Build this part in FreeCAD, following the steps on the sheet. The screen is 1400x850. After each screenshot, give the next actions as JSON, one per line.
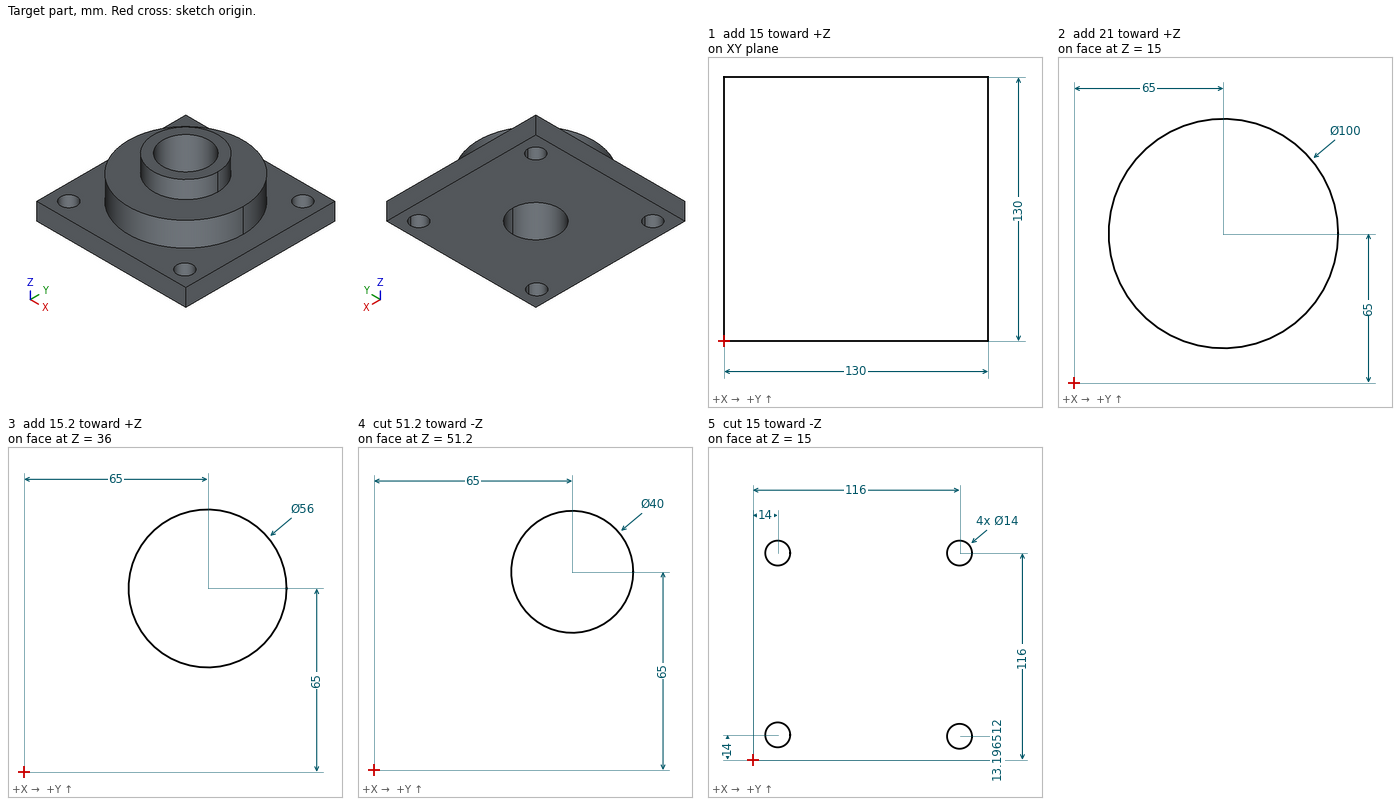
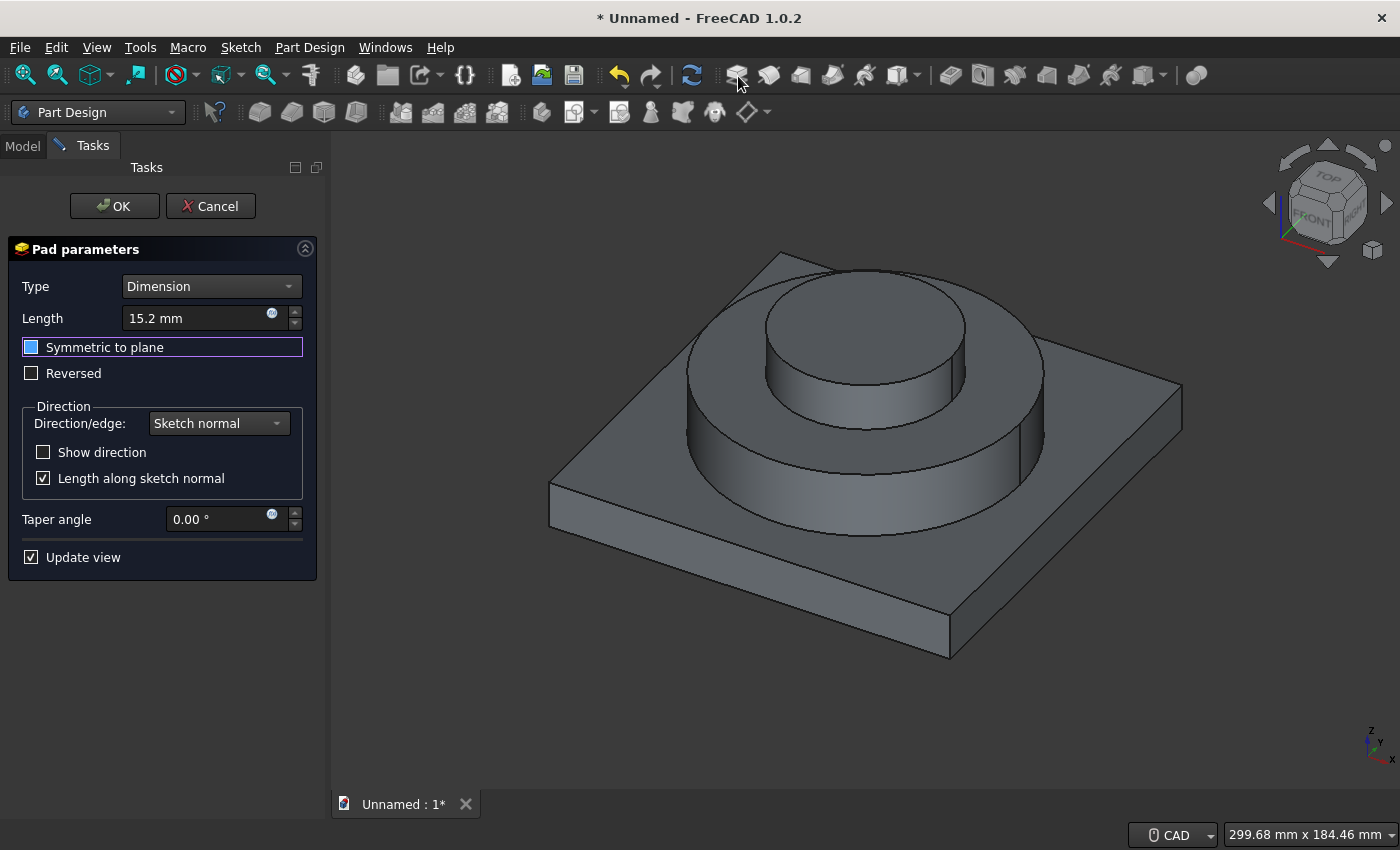
{"action": "left_click", "coordinate": [115, 206]}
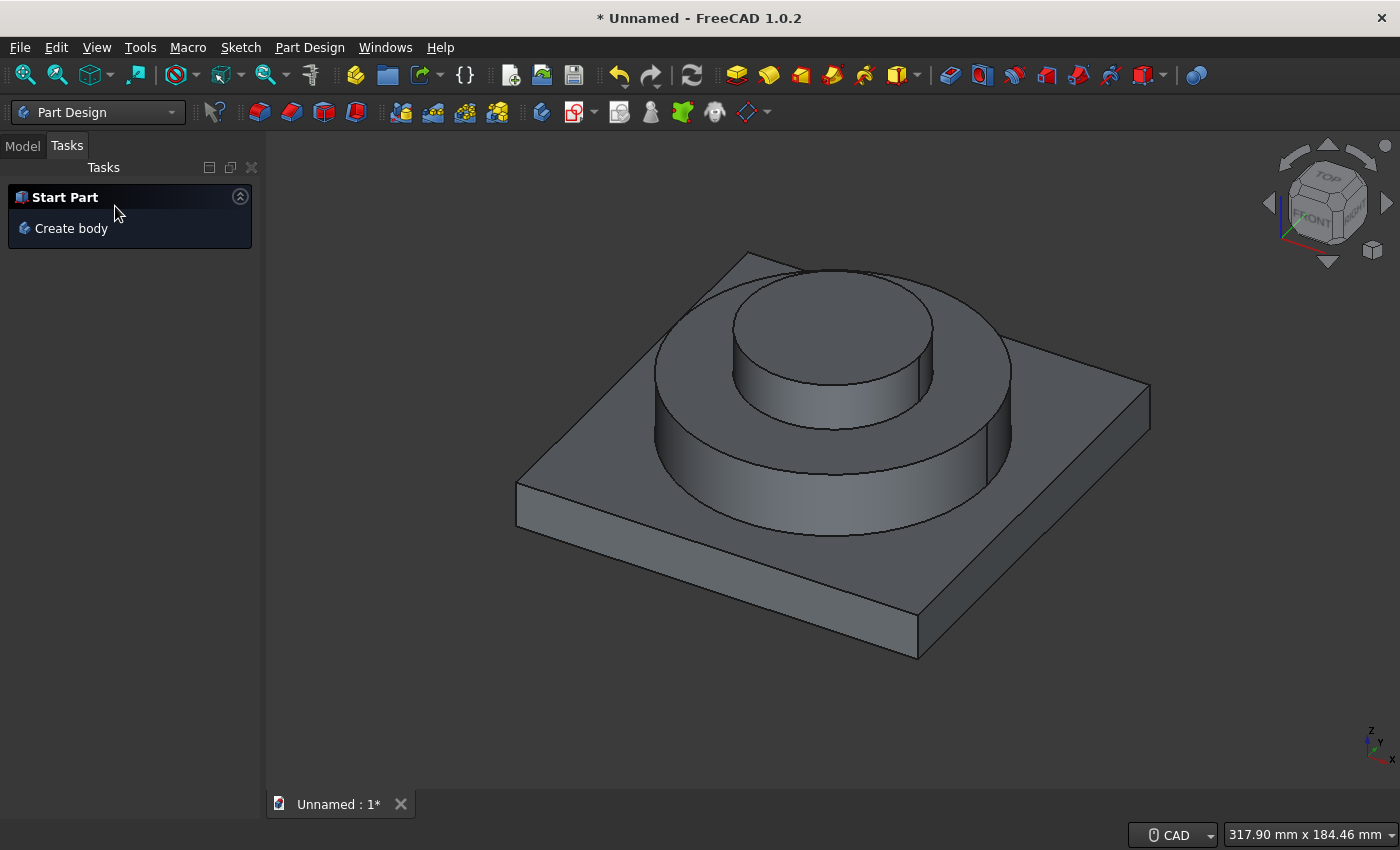
{"action": "left_click", "coordinate": [833, 327]}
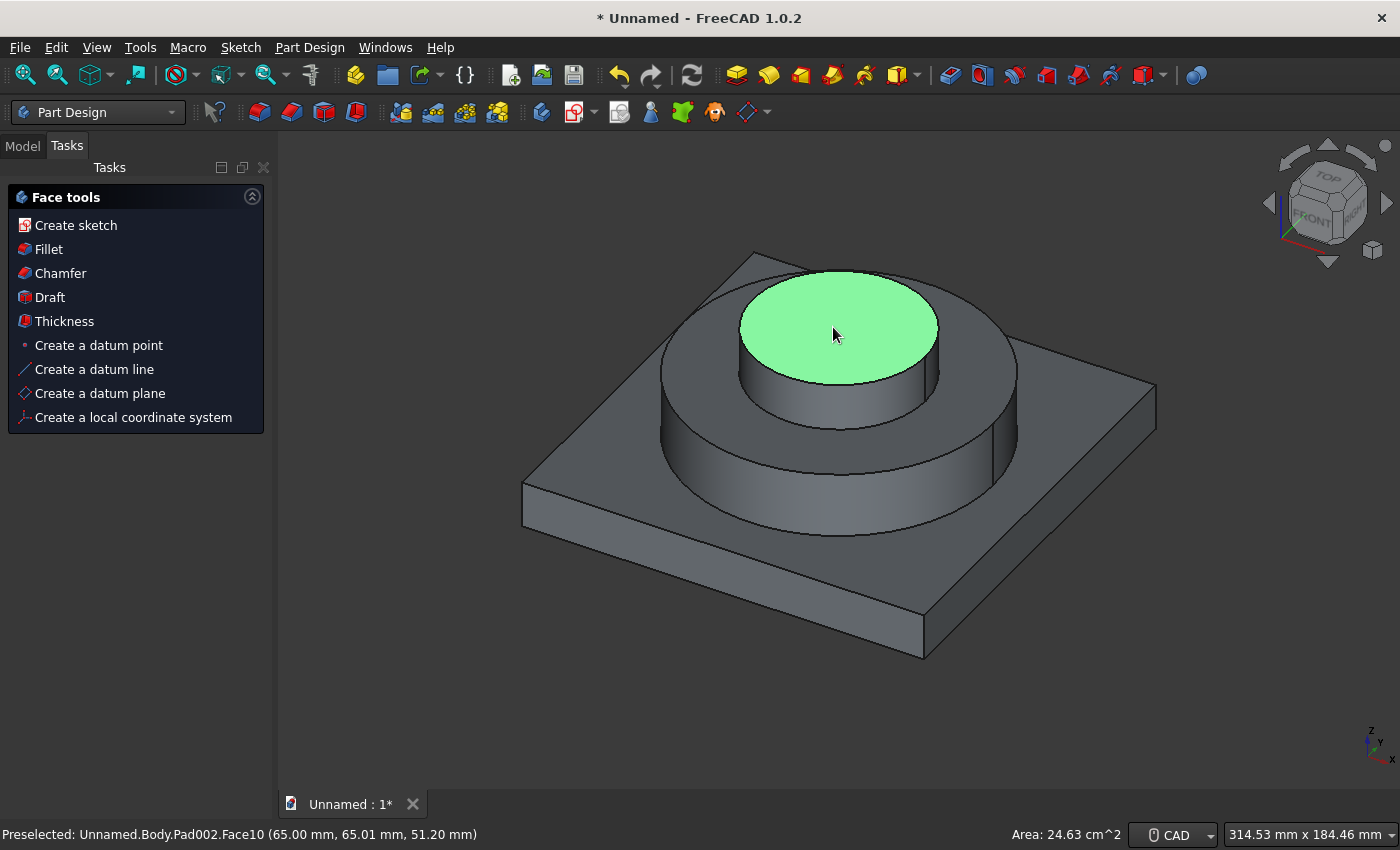
{"action": "left_click", "coordinate": [574, 112]}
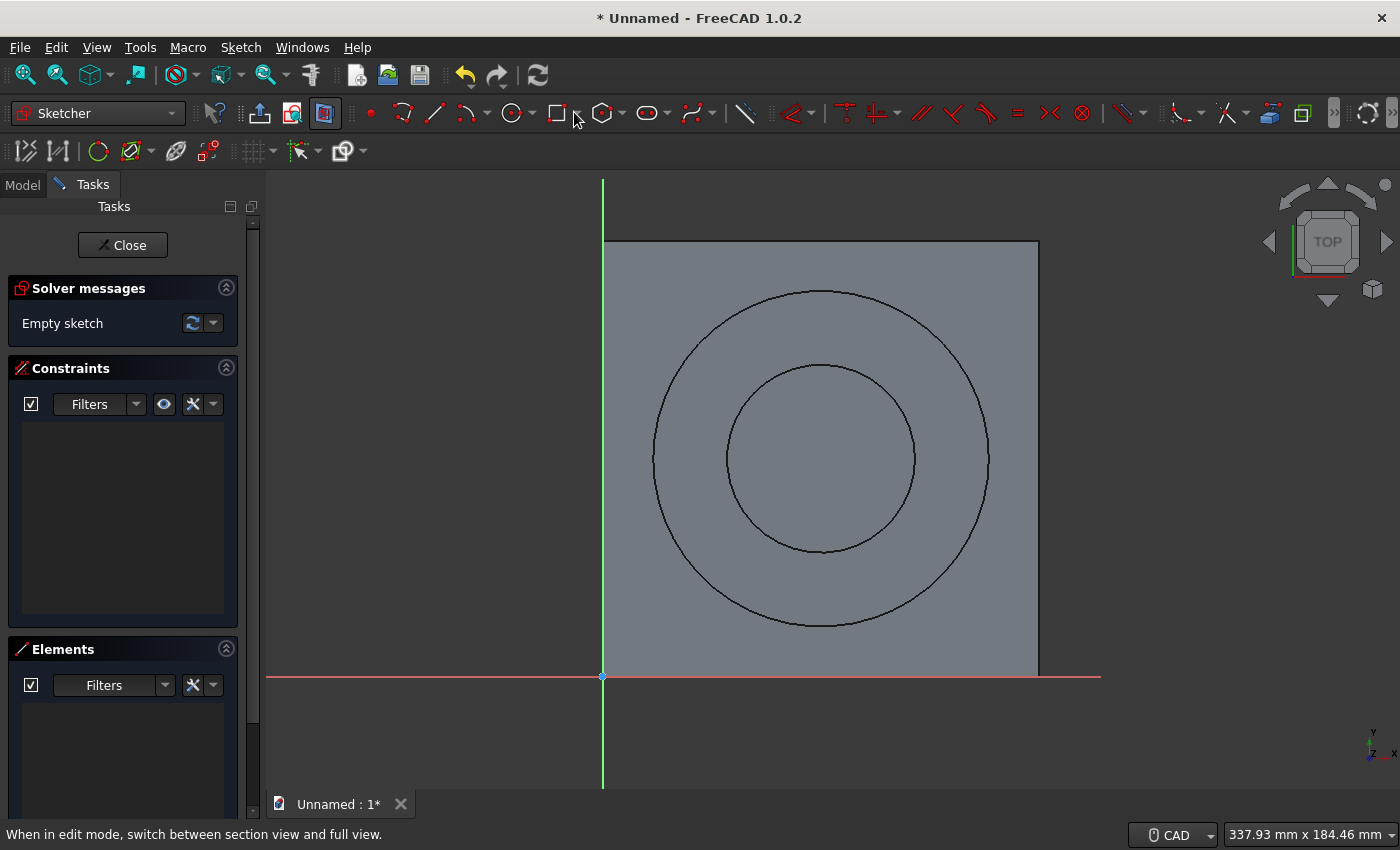
{"action": "scroll", "coordinate": [707, 646], "scroll_direction": "up", "scroll_amount": 2}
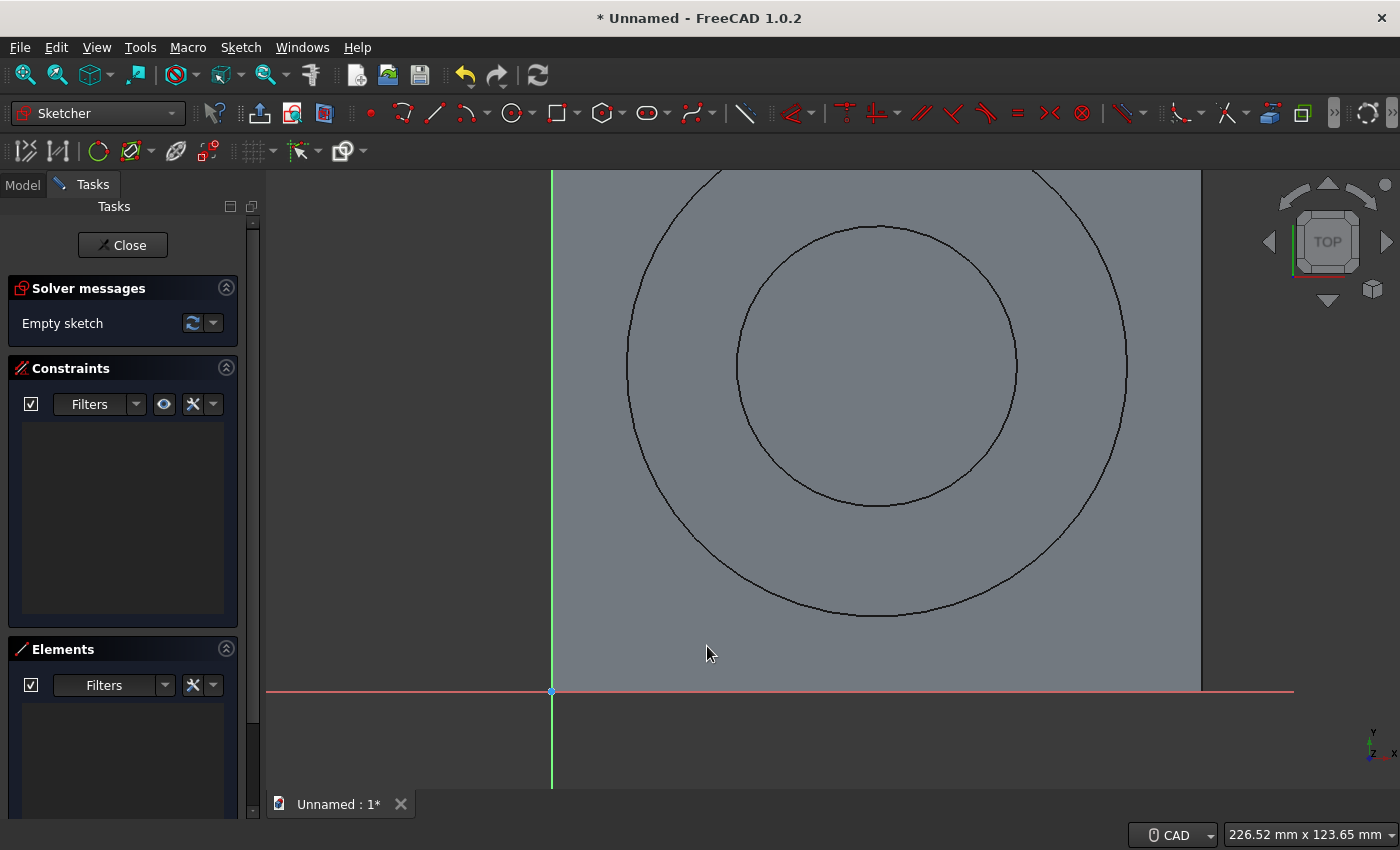
{"action": "key", "text": "g c"}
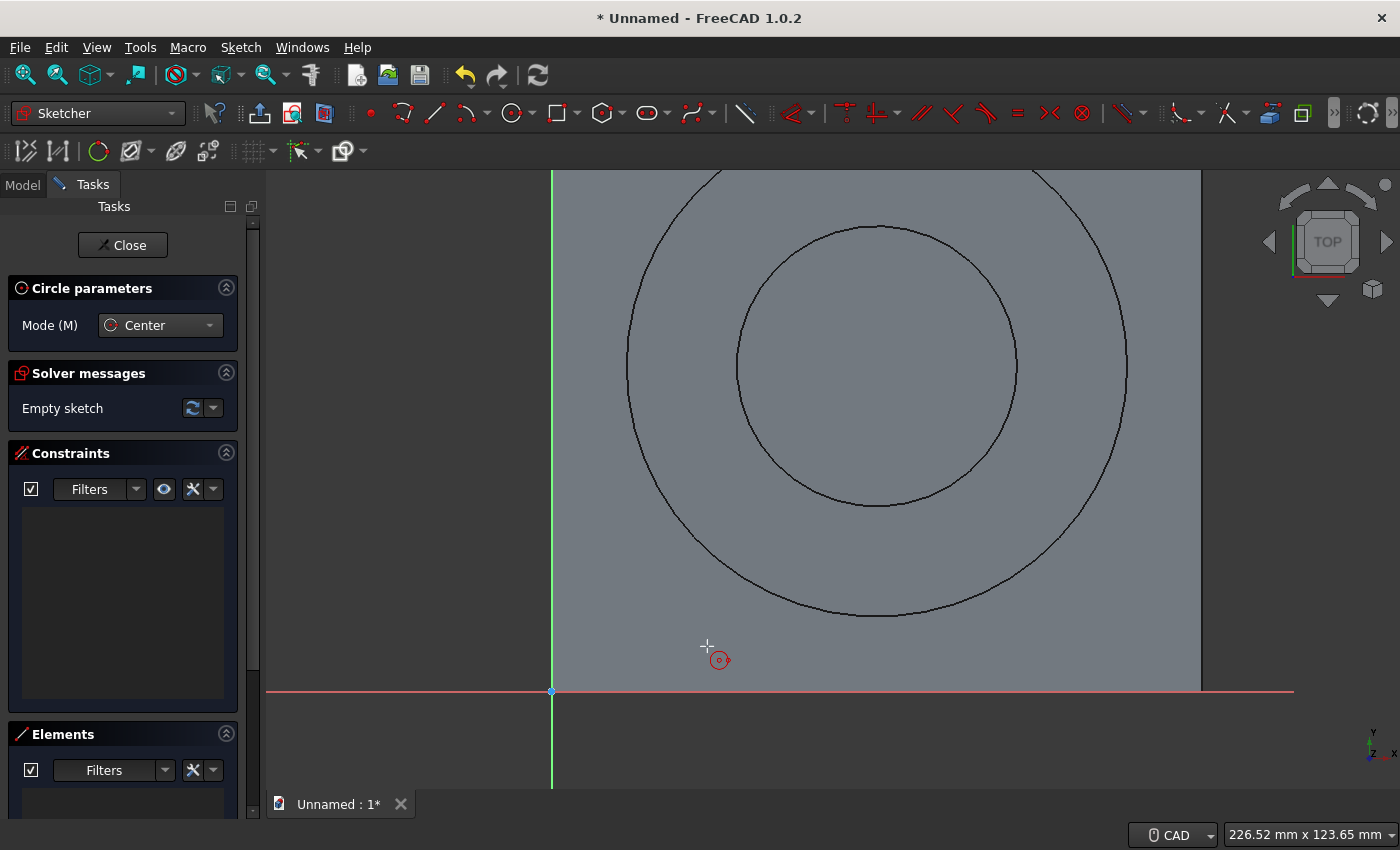
{"action": "left_click", "coordinate": [877, 366]}
{"action": "mouse_move", "coordinate": [948, 296]}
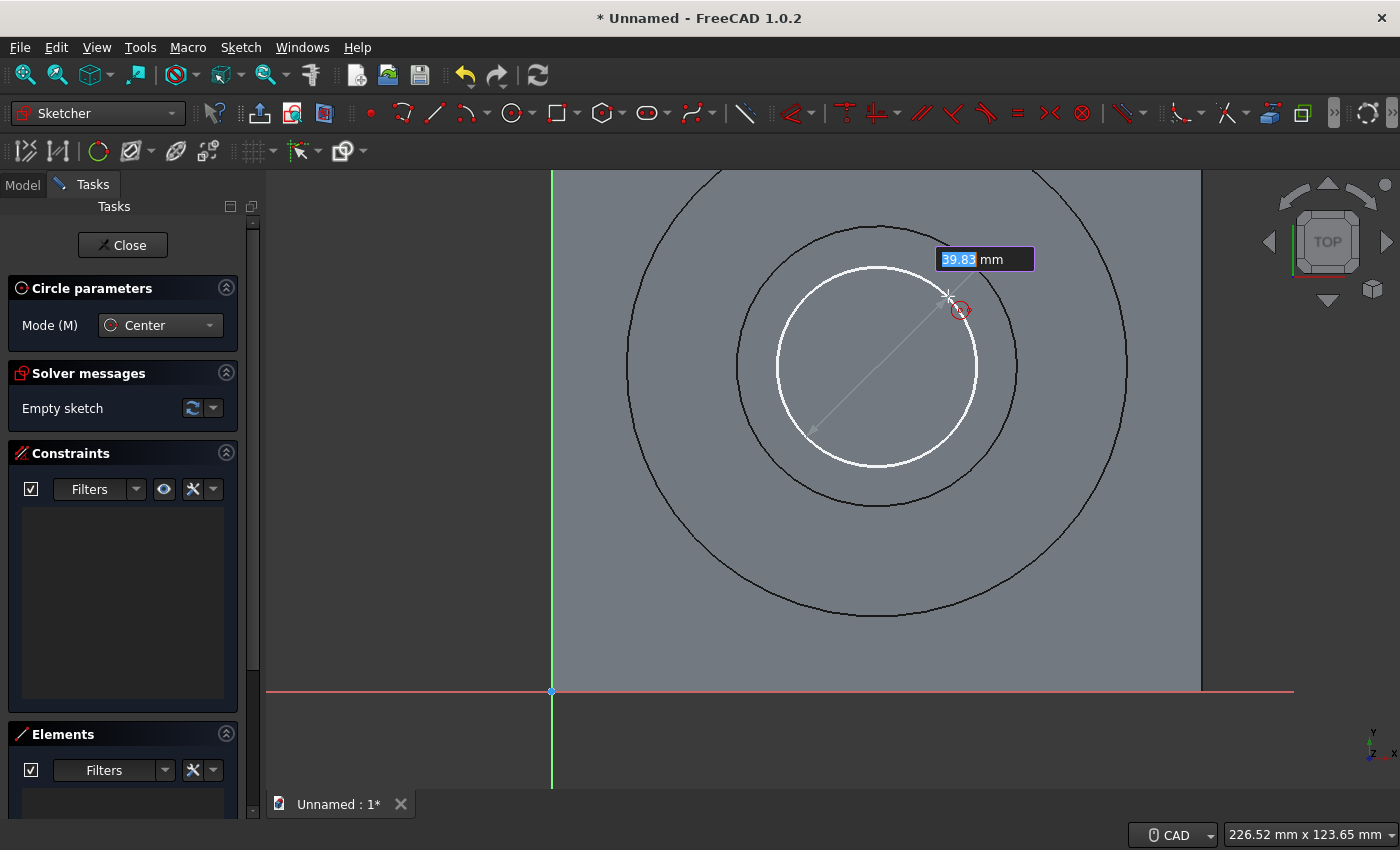
{"action": "type", "text": "40"}
{"action": "key", "text": "Return"}
{"action": "key", "text": "Escape"}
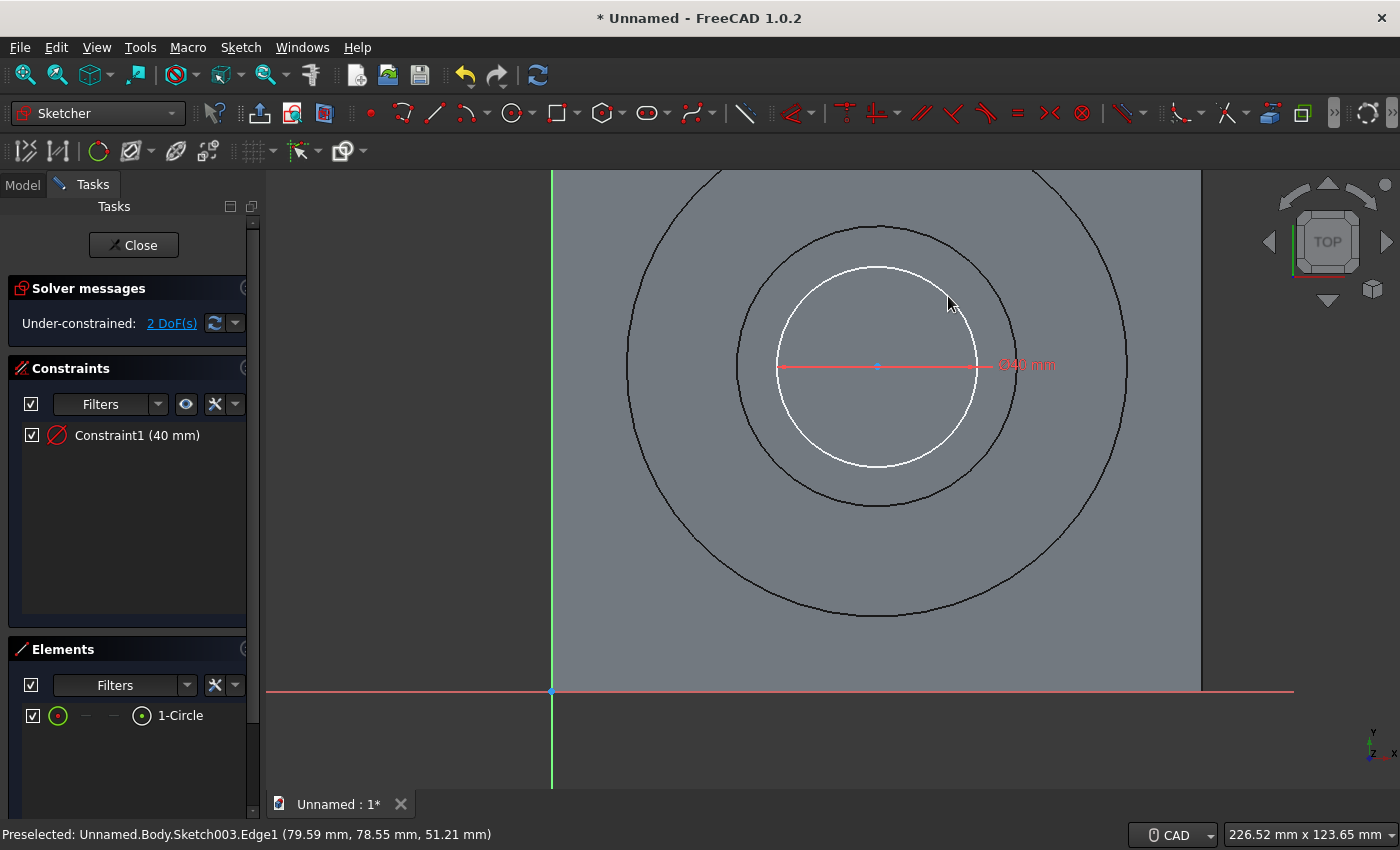
{"action": "key", "text": "d"}